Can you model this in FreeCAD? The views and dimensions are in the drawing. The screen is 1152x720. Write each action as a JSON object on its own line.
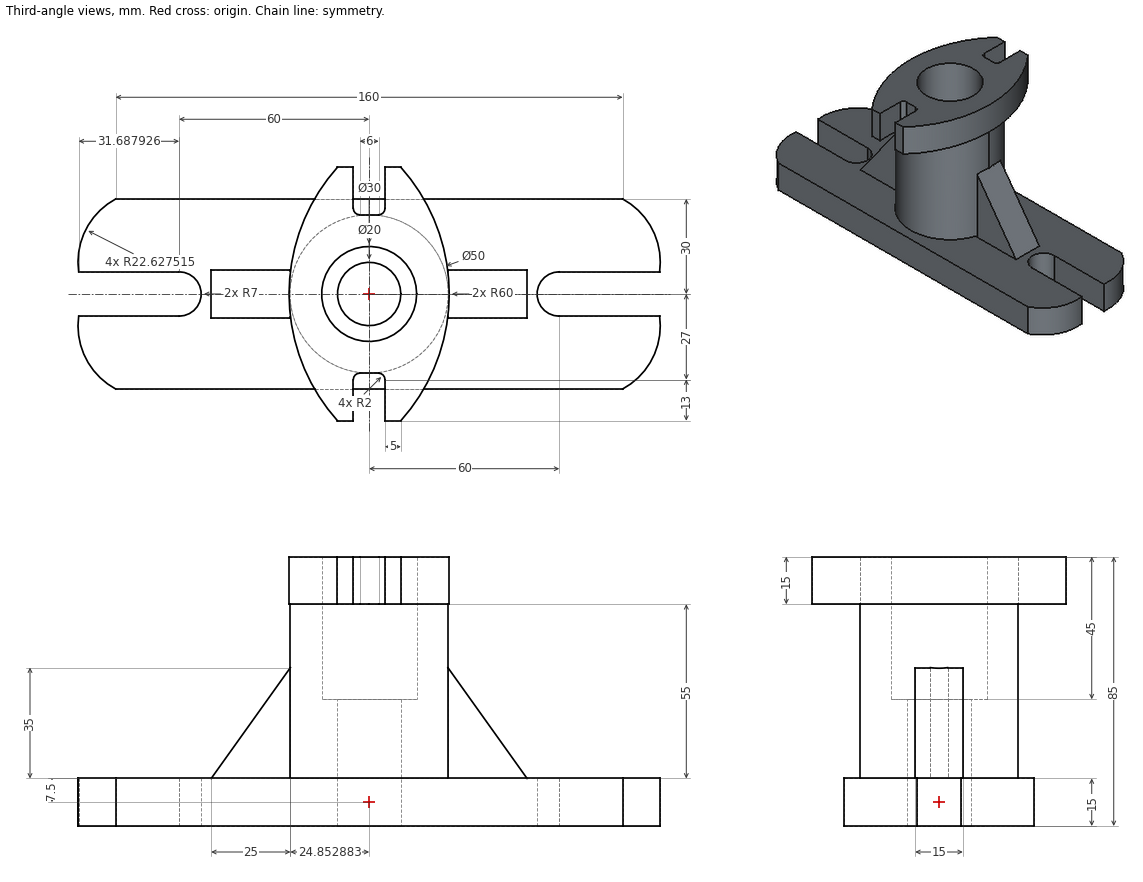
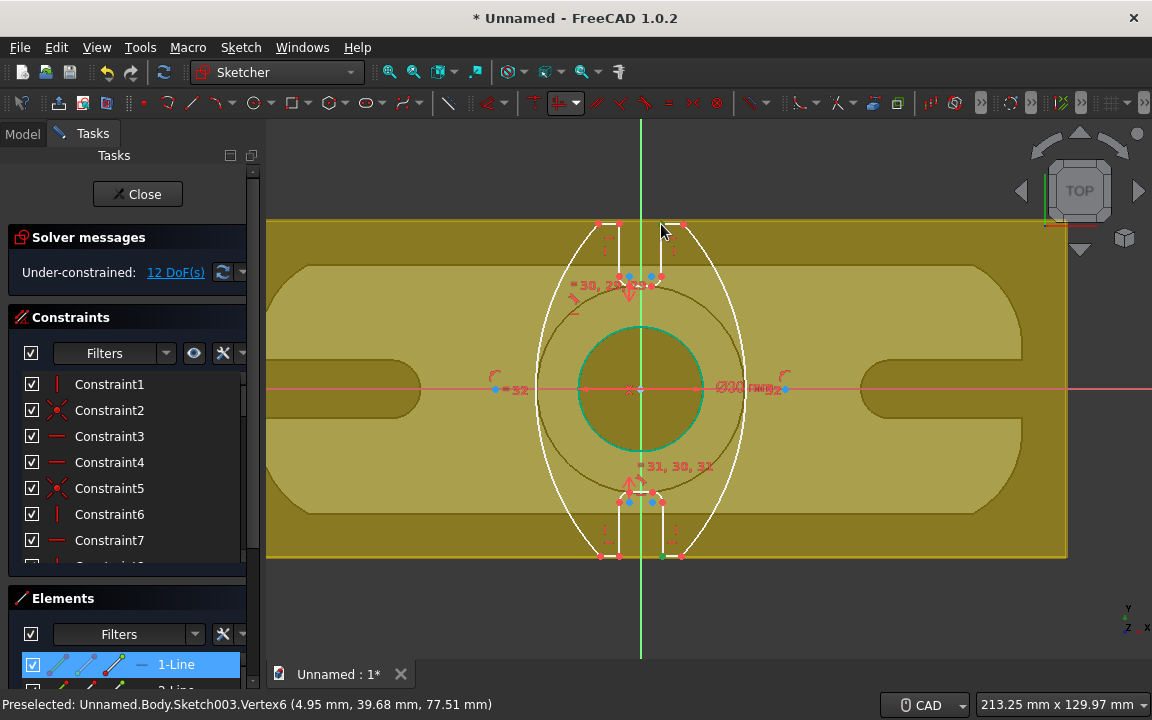
{"action": "left_click", "coordinate": [344, 389]}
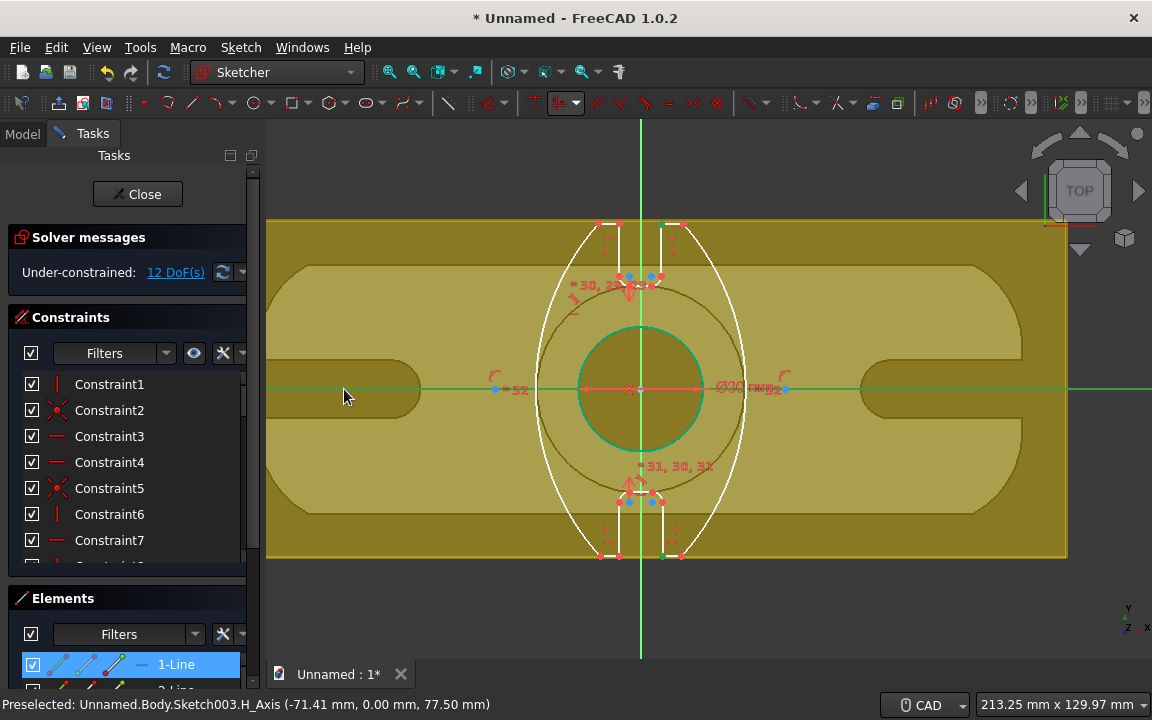
{"action": "key", "text": "s"}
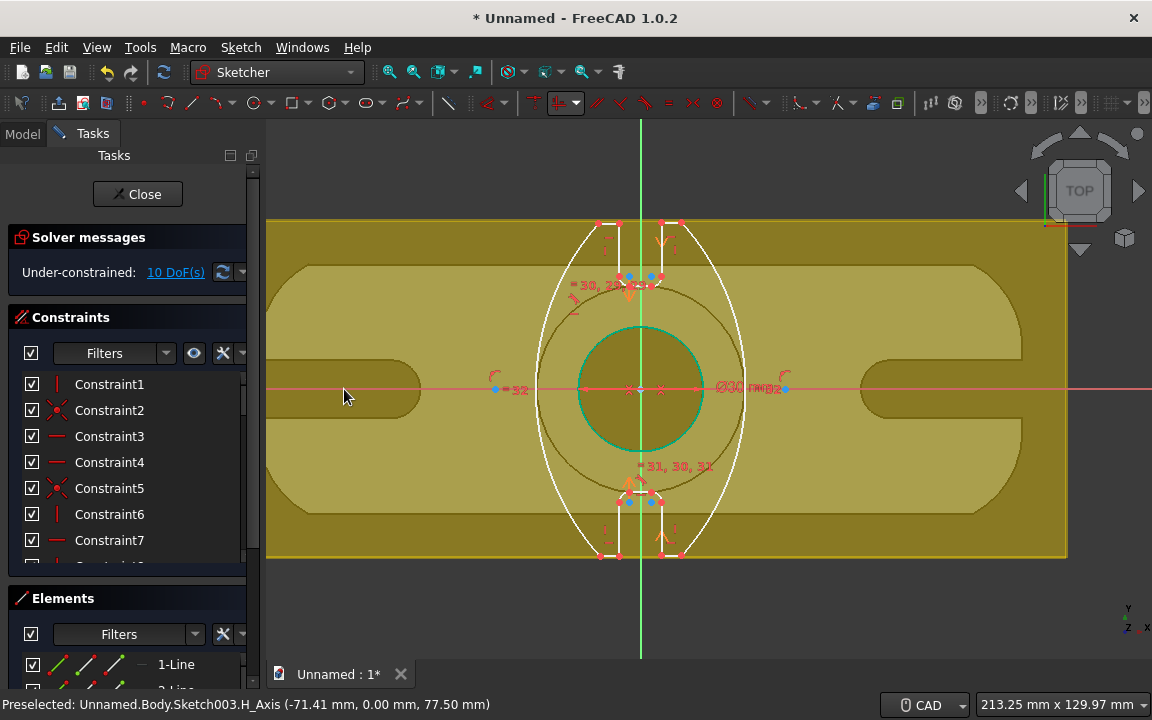
{"action": "left_click", "coordinate": [662, 223]}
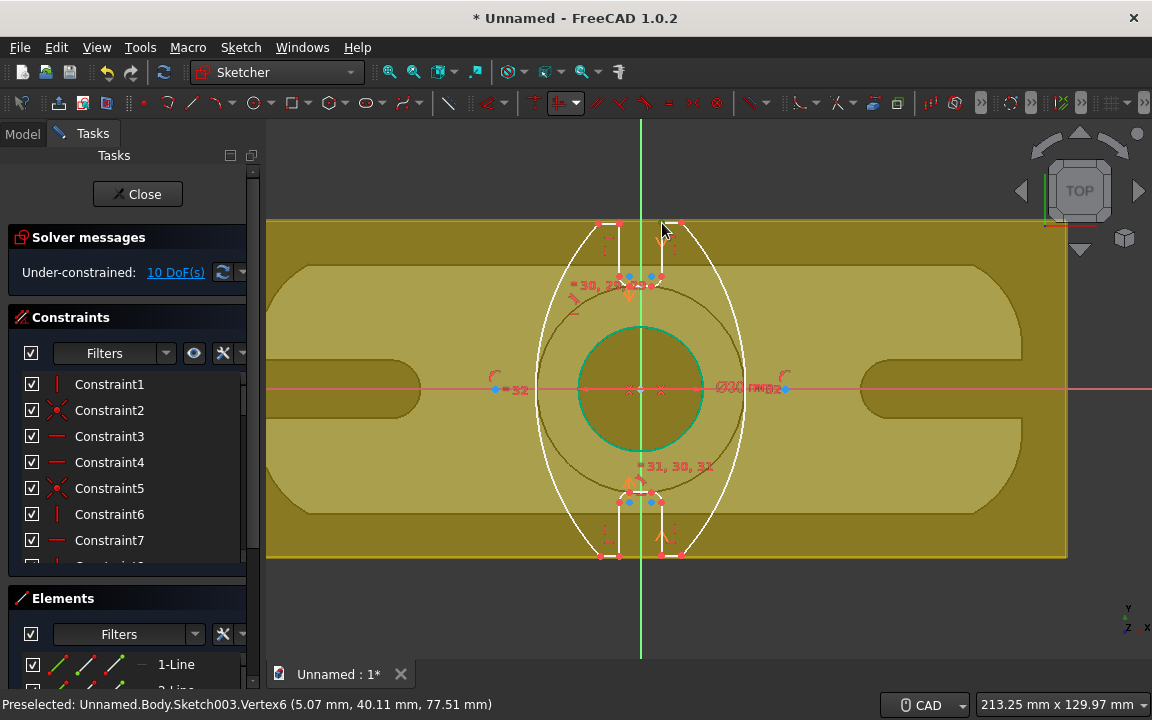
{"action": "left_click", "coordinate": [619, 224]}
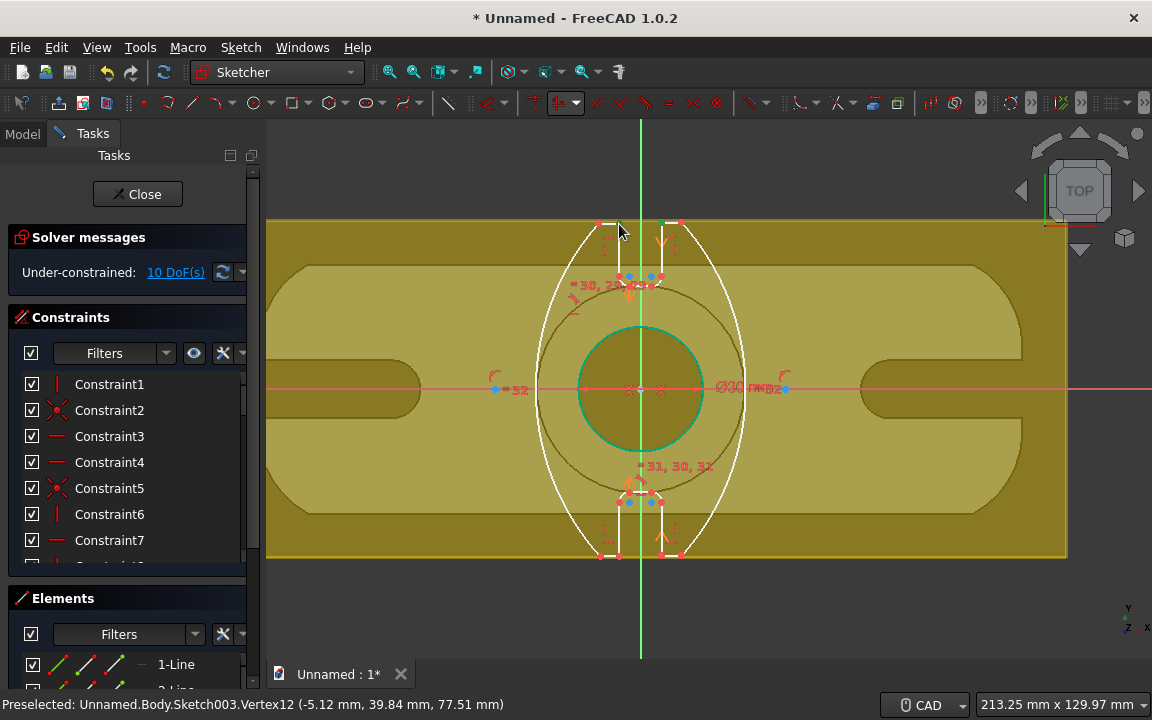
{"action": "left_click", "coordinate": [641, 596]}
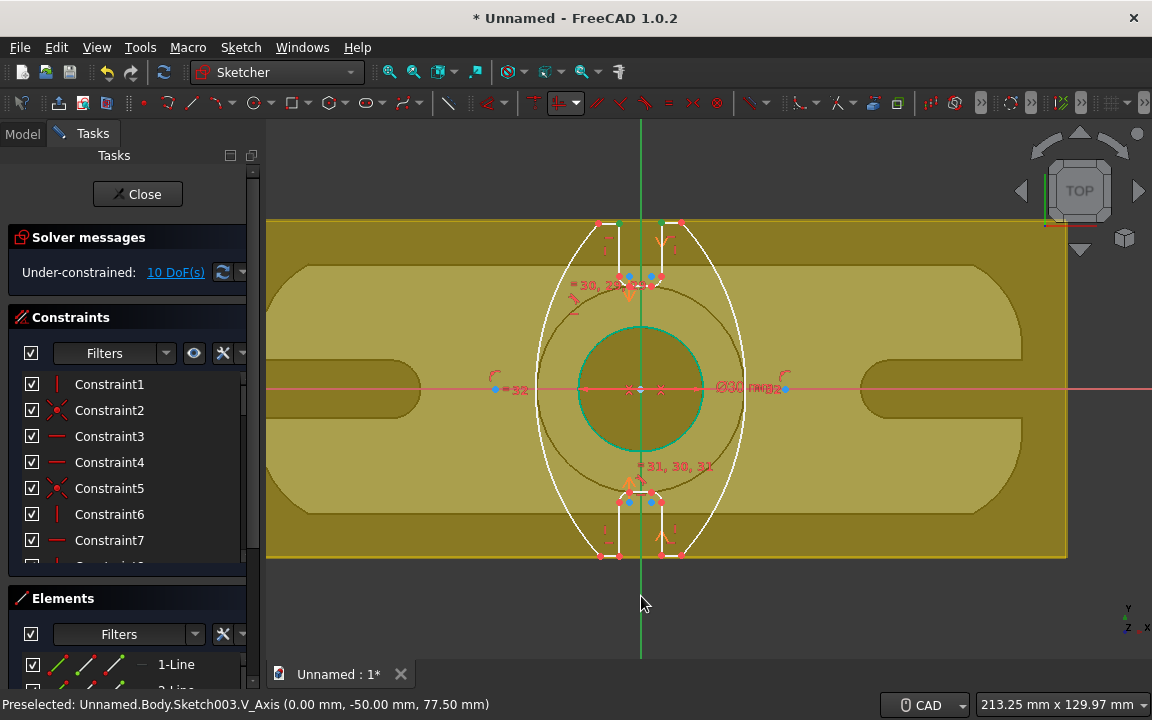
{"action": "key", "text": "s"}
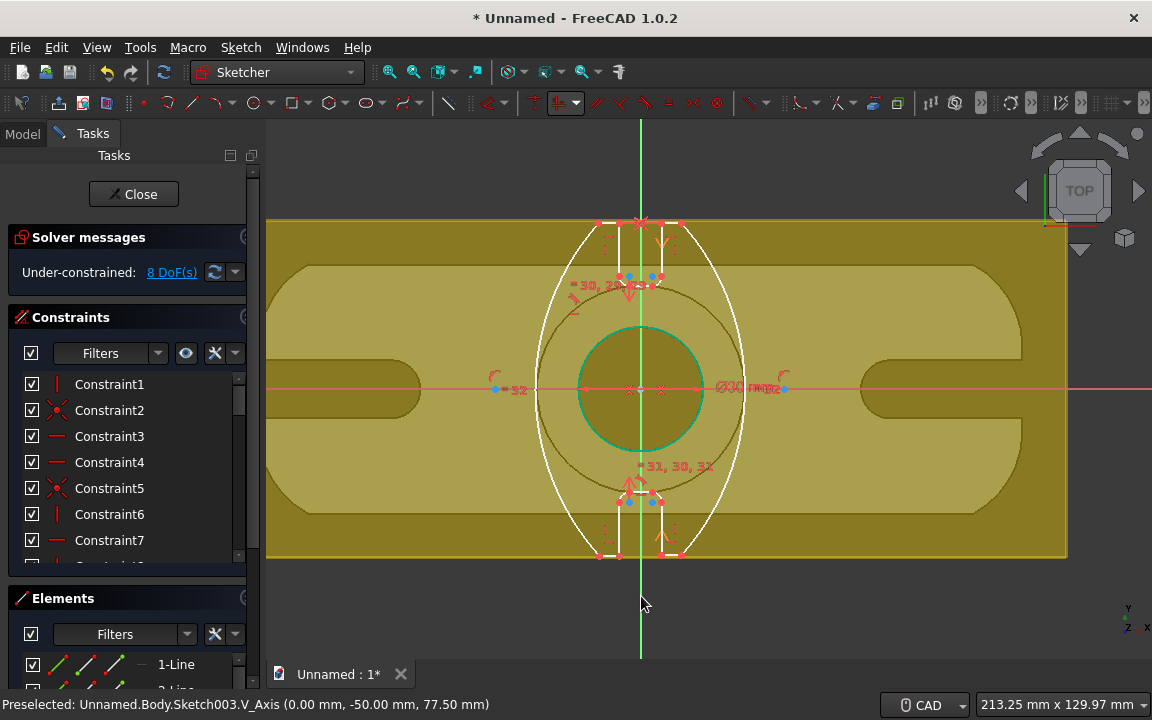
{"action": "left_click", "coordinate": [682, 555]}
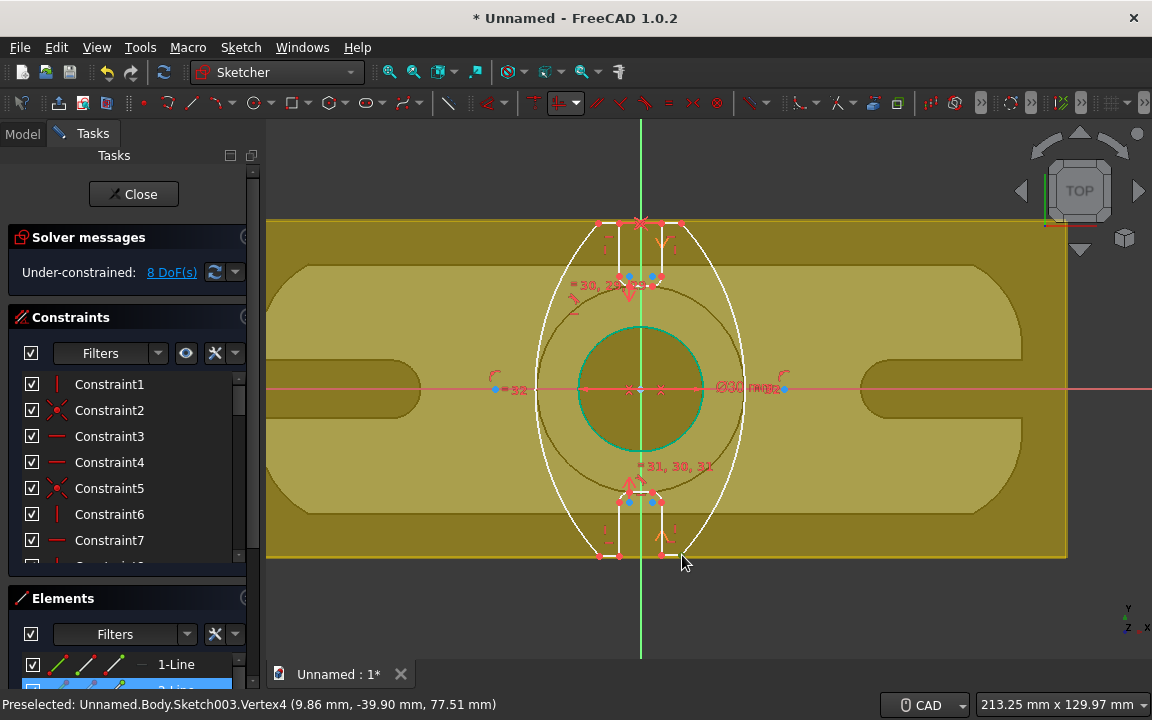
{"action": "left_click", "coordinate": [600, 556]}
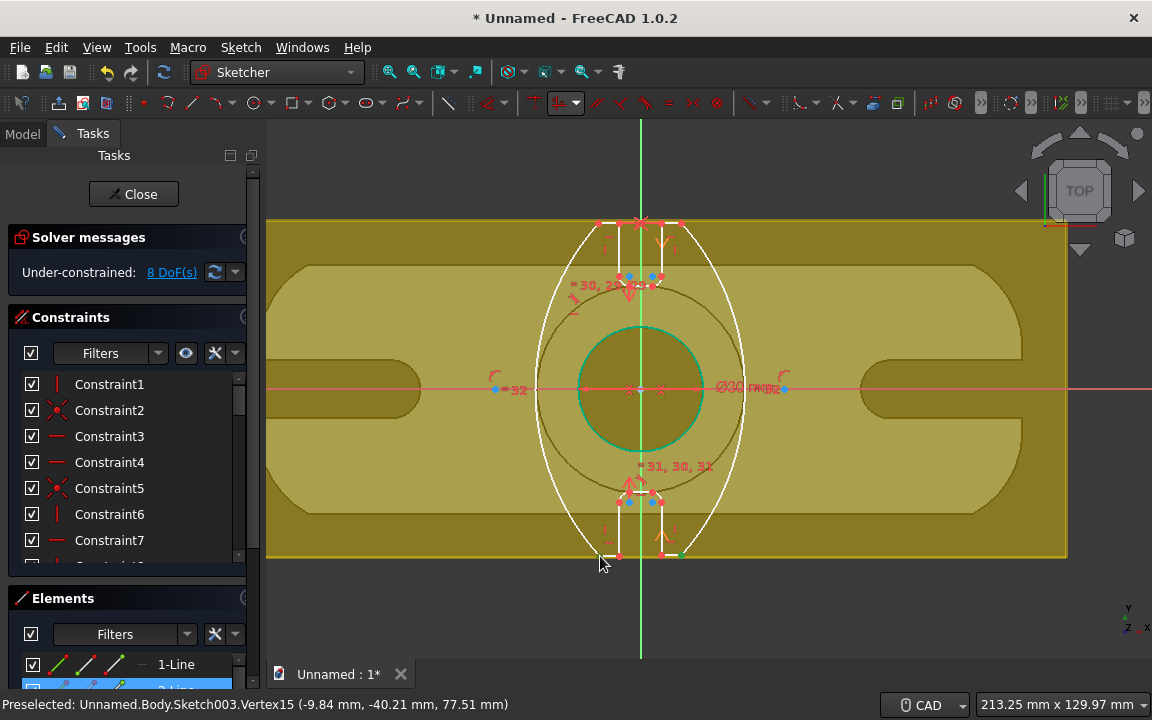
{"action": "left_click", "coordinate": [641, 596]}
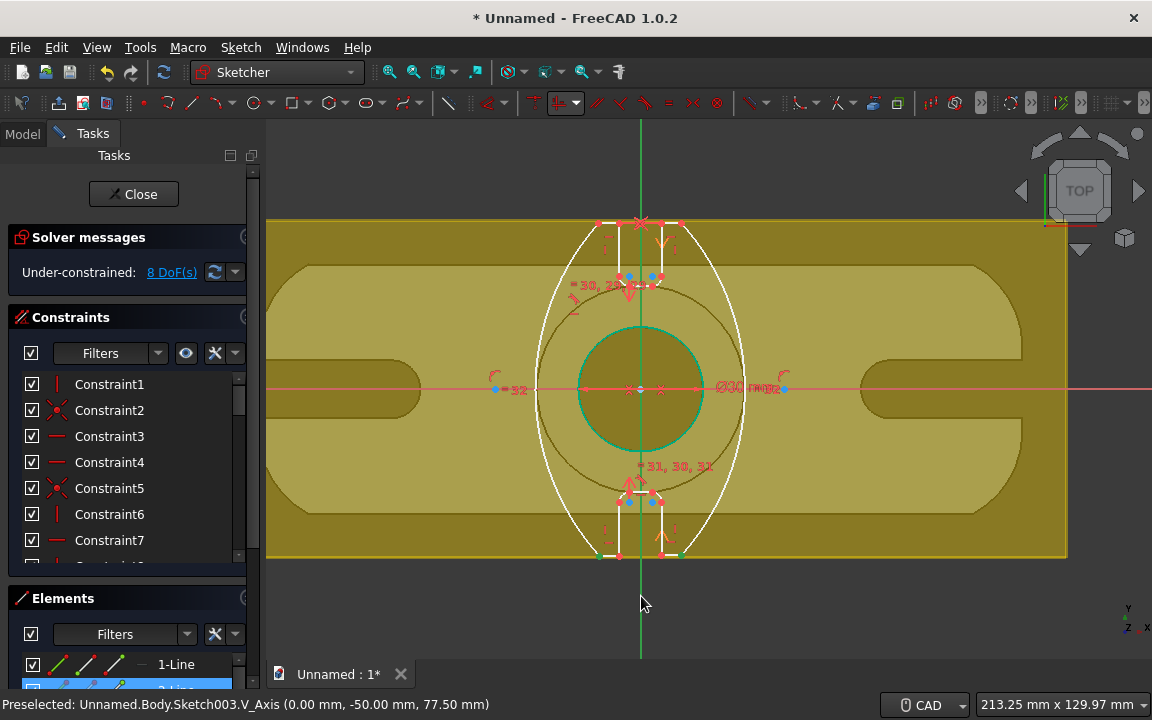
{"action": "key", "text": "s"}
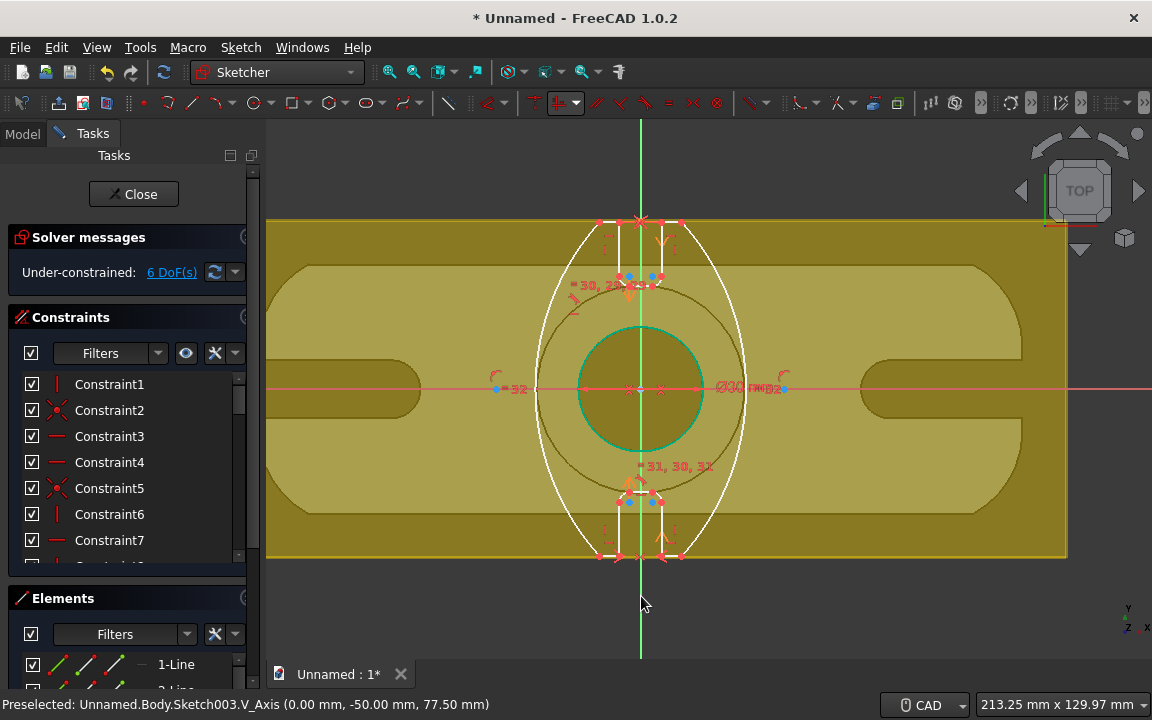
{"action": "key", "text": "d"}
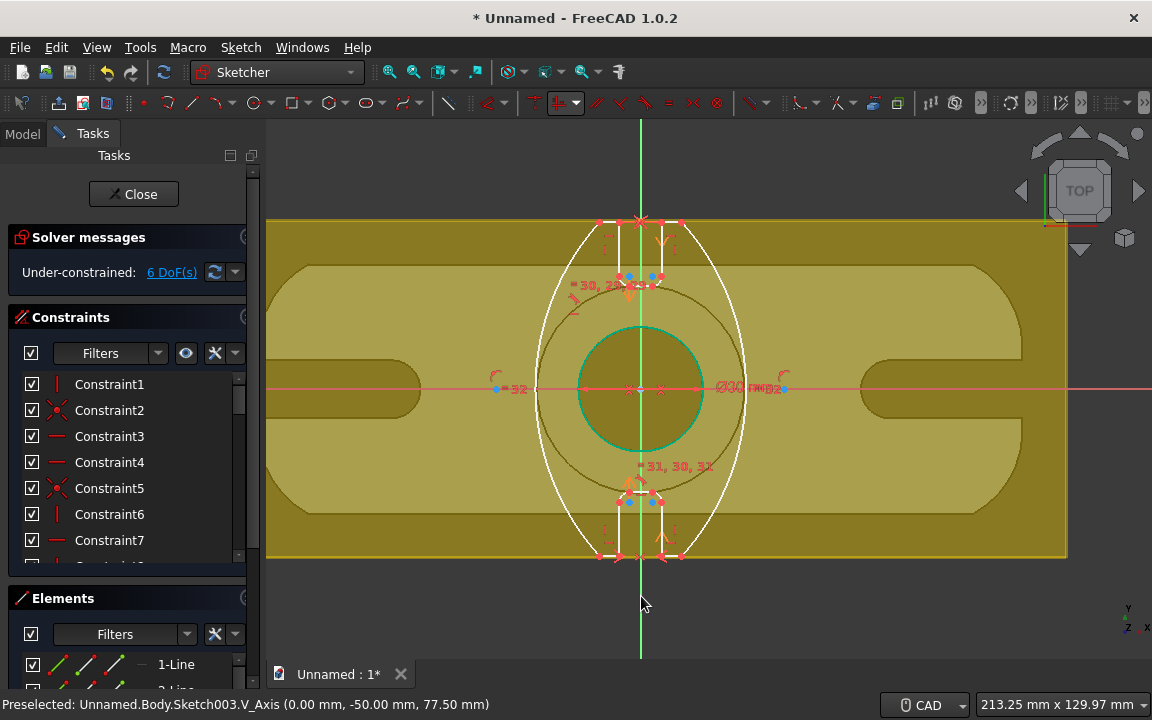
{"action": "left_click", "coordinate": [735, 461]}
{"action": "left_click", "coordinate": [766, 470]}